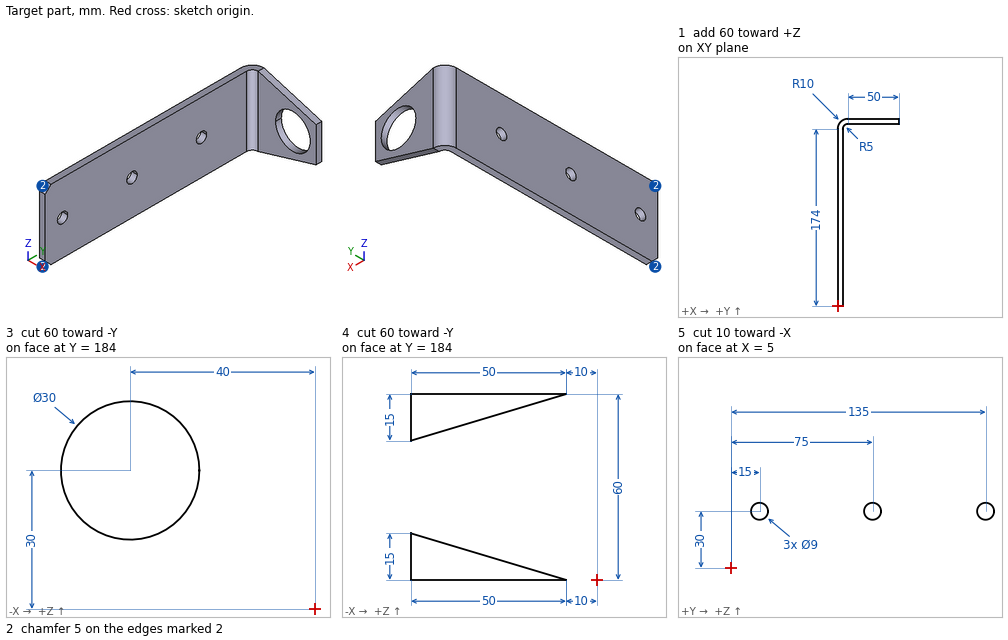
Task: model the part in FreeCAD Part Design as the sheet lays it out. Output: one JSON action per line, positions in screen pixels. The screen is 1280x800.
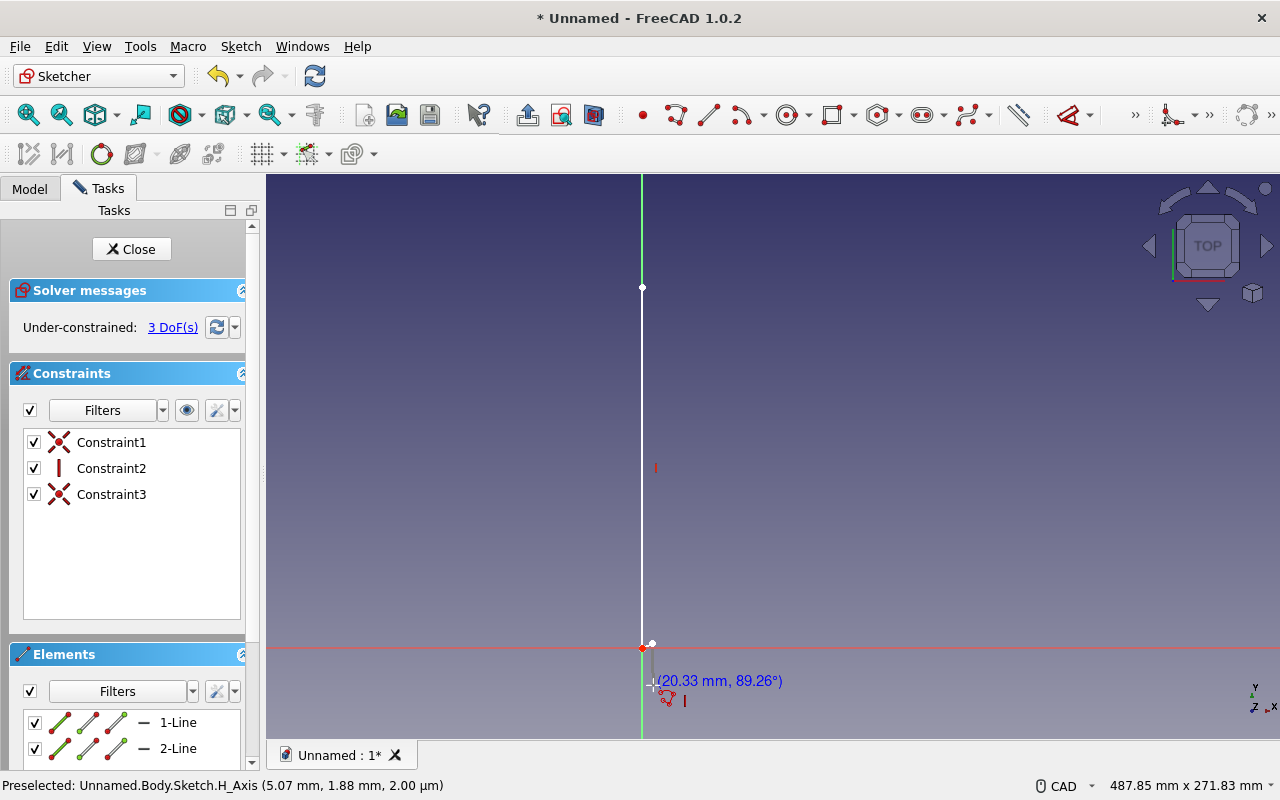
{"action": "scroll", "coordinate": [653, 287], "scroll_direction": "up", "scroll_amount": 3}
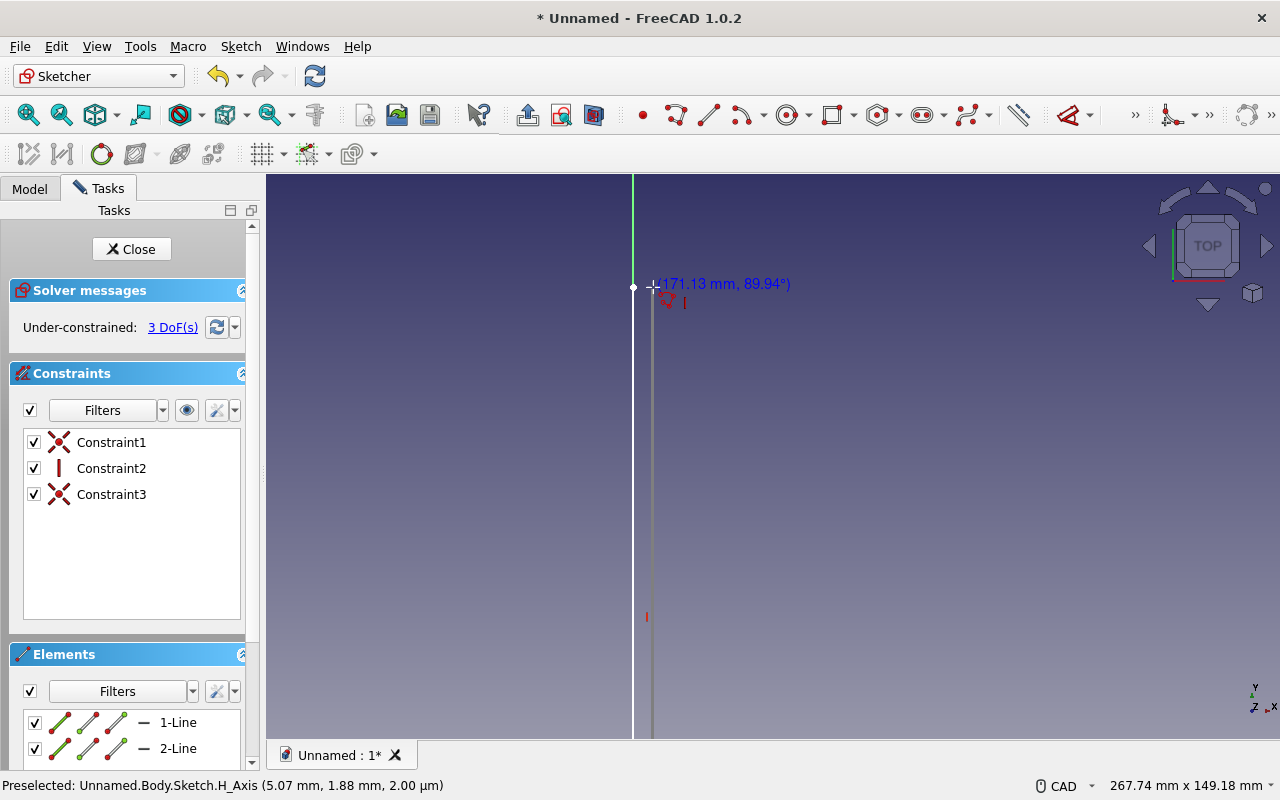
{"action": "left_click", "coordinate": [652, 286]}
{"action": "right_click", "coordinate": [652, 286]}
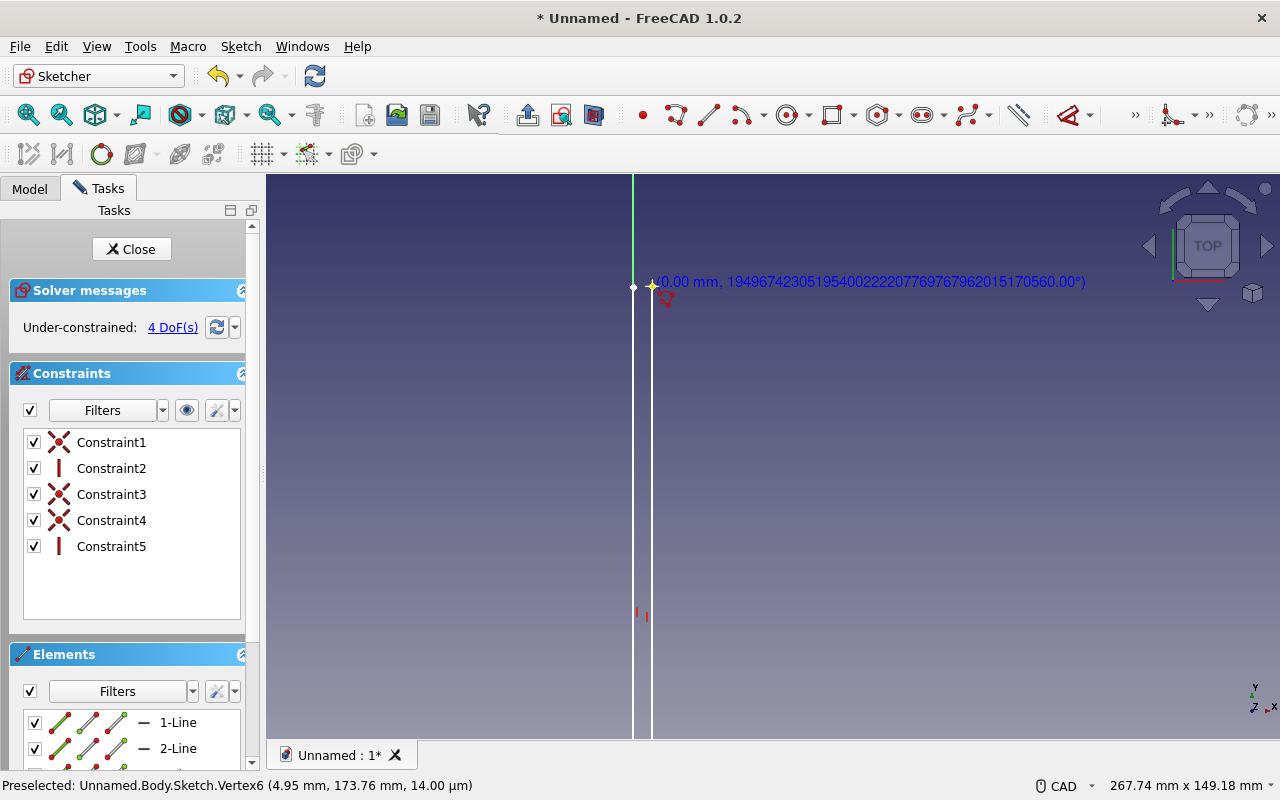
{"action": "left_click", "coordinate": [671, 267]}
{"action": "left_click", "coordinate": [860, 267]}
{"action": "left_click", "coordinate": [860, 248]}
{"action": "left_click", "coordinate": [671, 248]}
{"action": "right_click", "coordinate": [671, 248]}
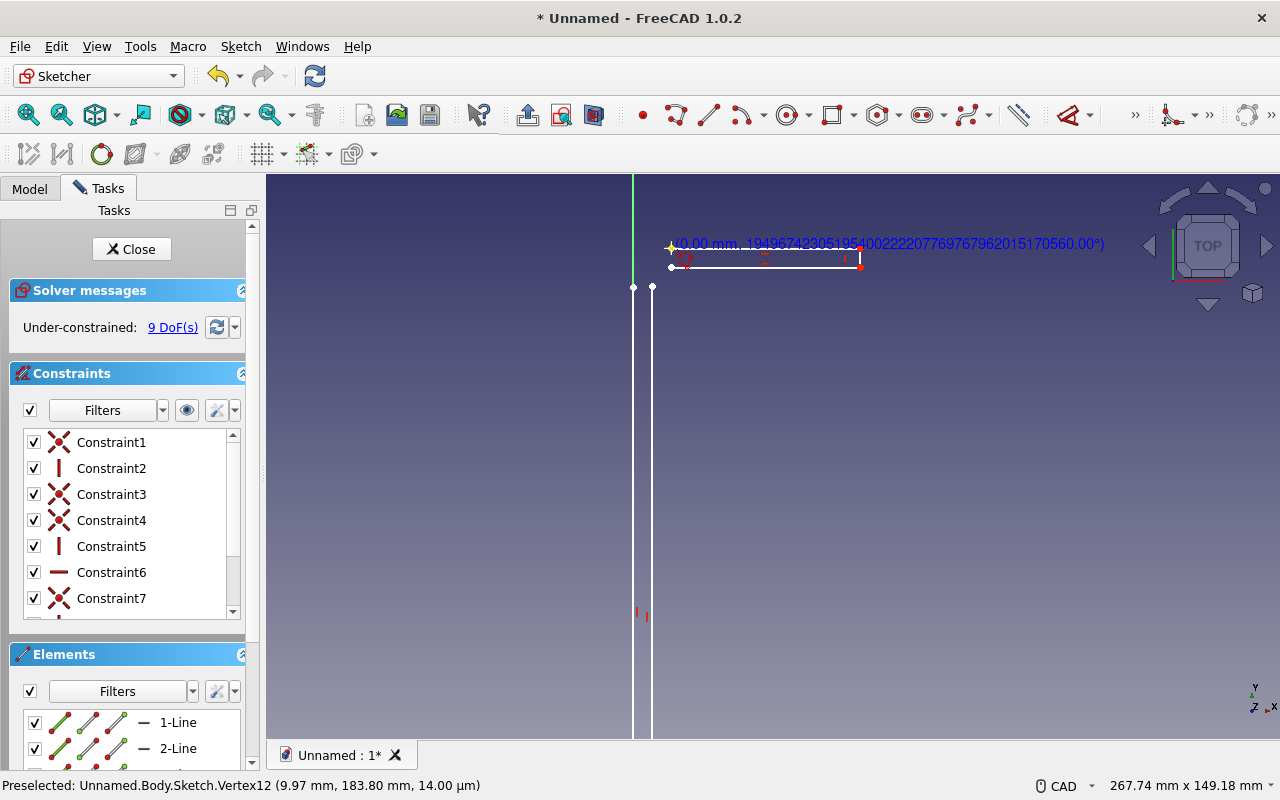
{"action": "key", "text": "g 3 a"}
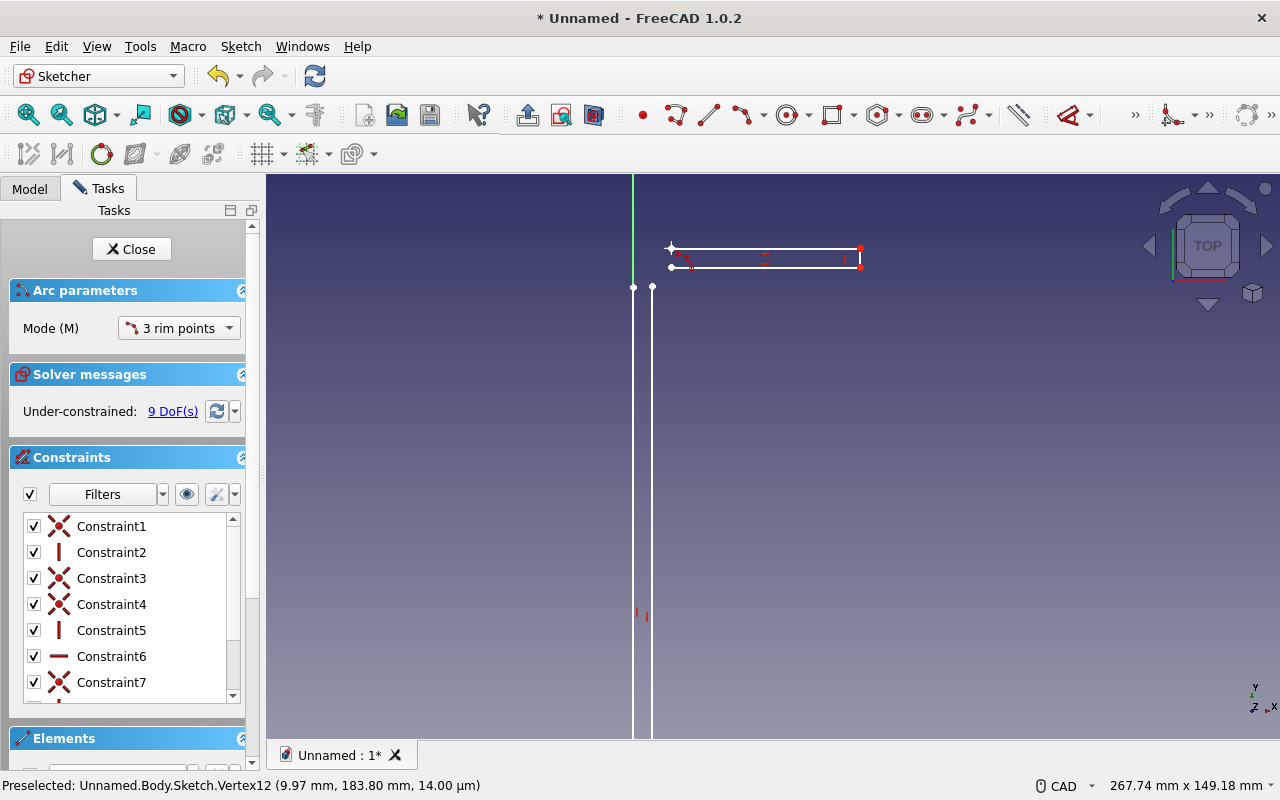
{"action": "left_click", "coordinate": [652, 287]}
{"action": "left_click", "coordinate": [671, 268]}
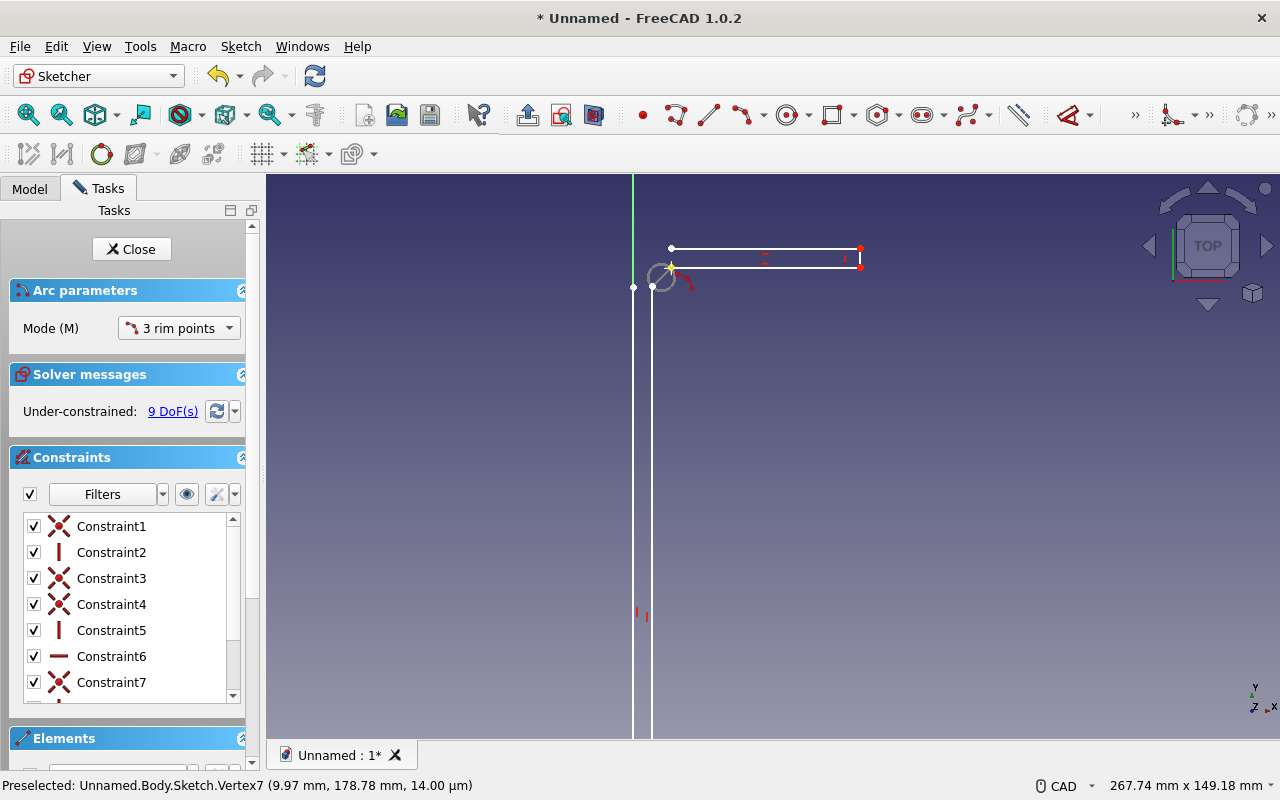
{"action": "scroll", "coordinate": [658, 273], "scroll_direction": "up", "scroll_amount": 6}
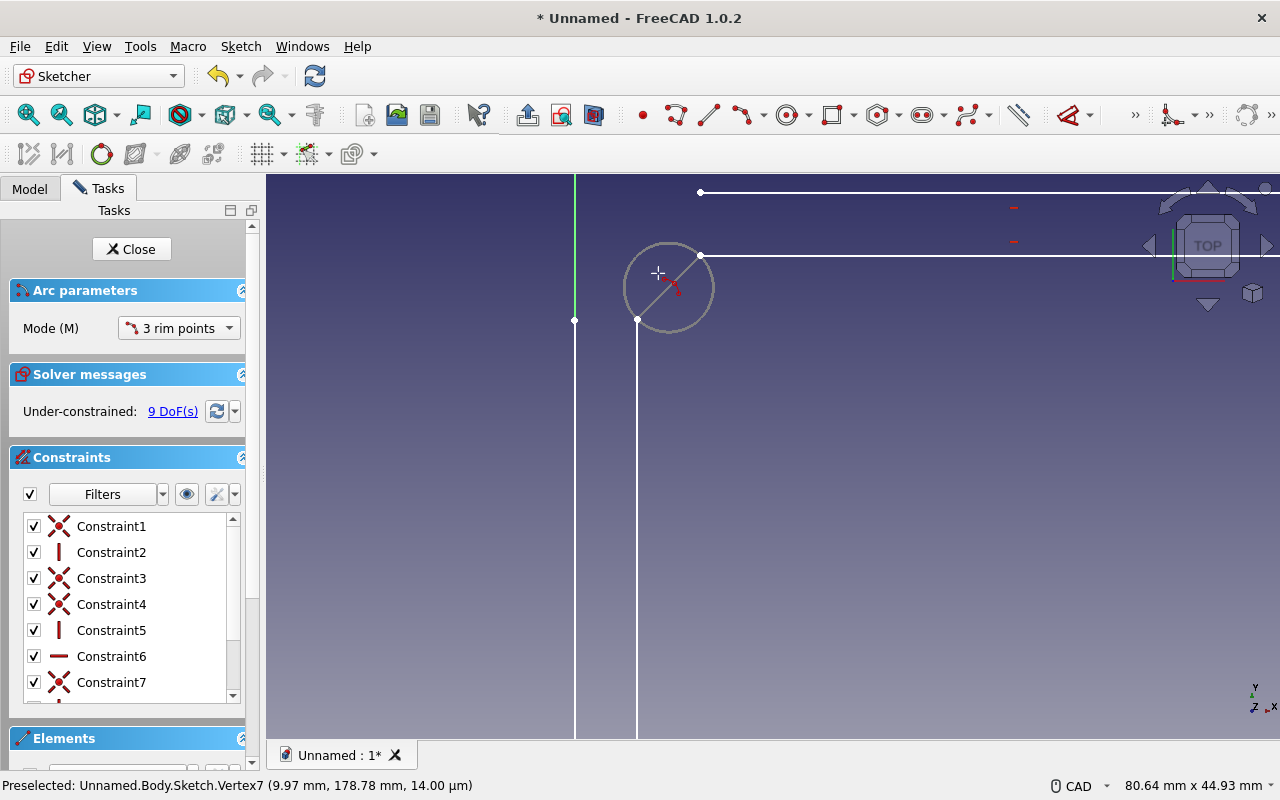
{"action": "left_click", "coordinate": [656, 272]}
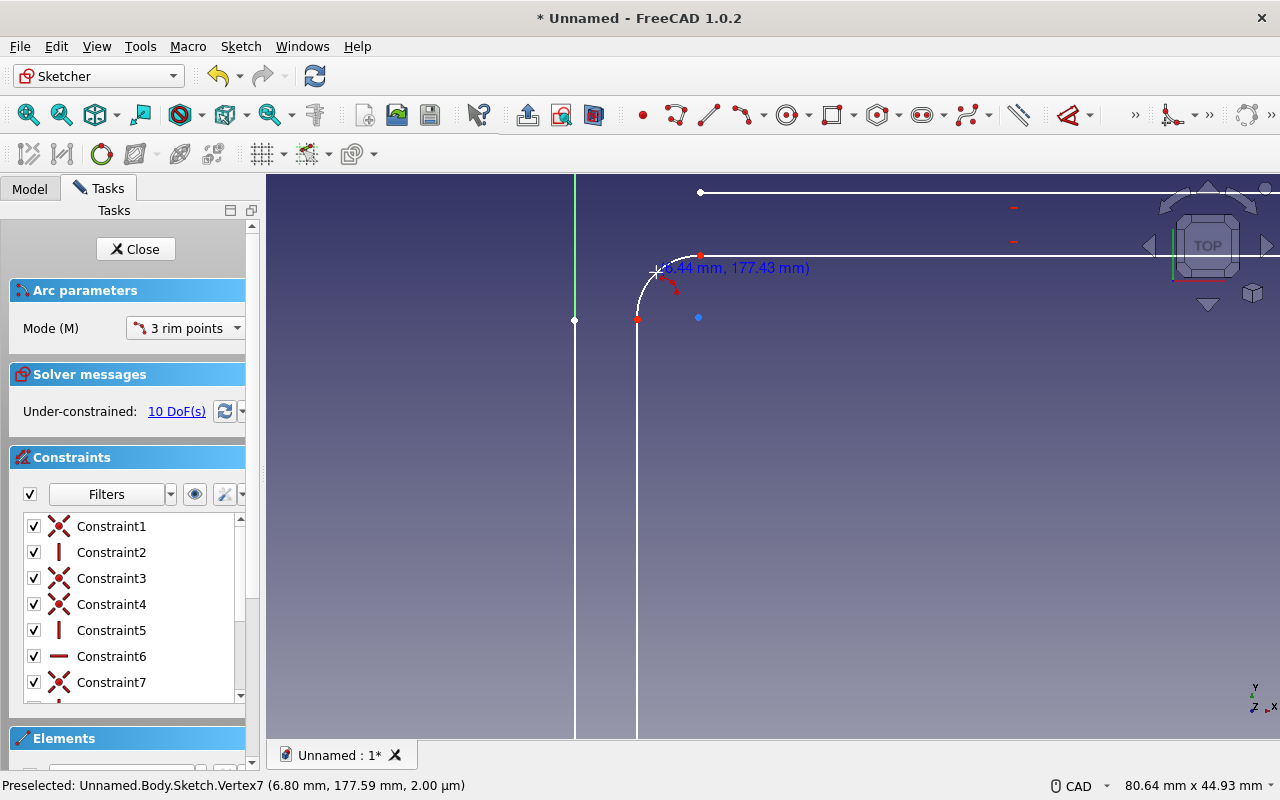
{"action": "scroll", "coordinate": [655, 280], "scroll_direction": "down", "scroll_amount": 9}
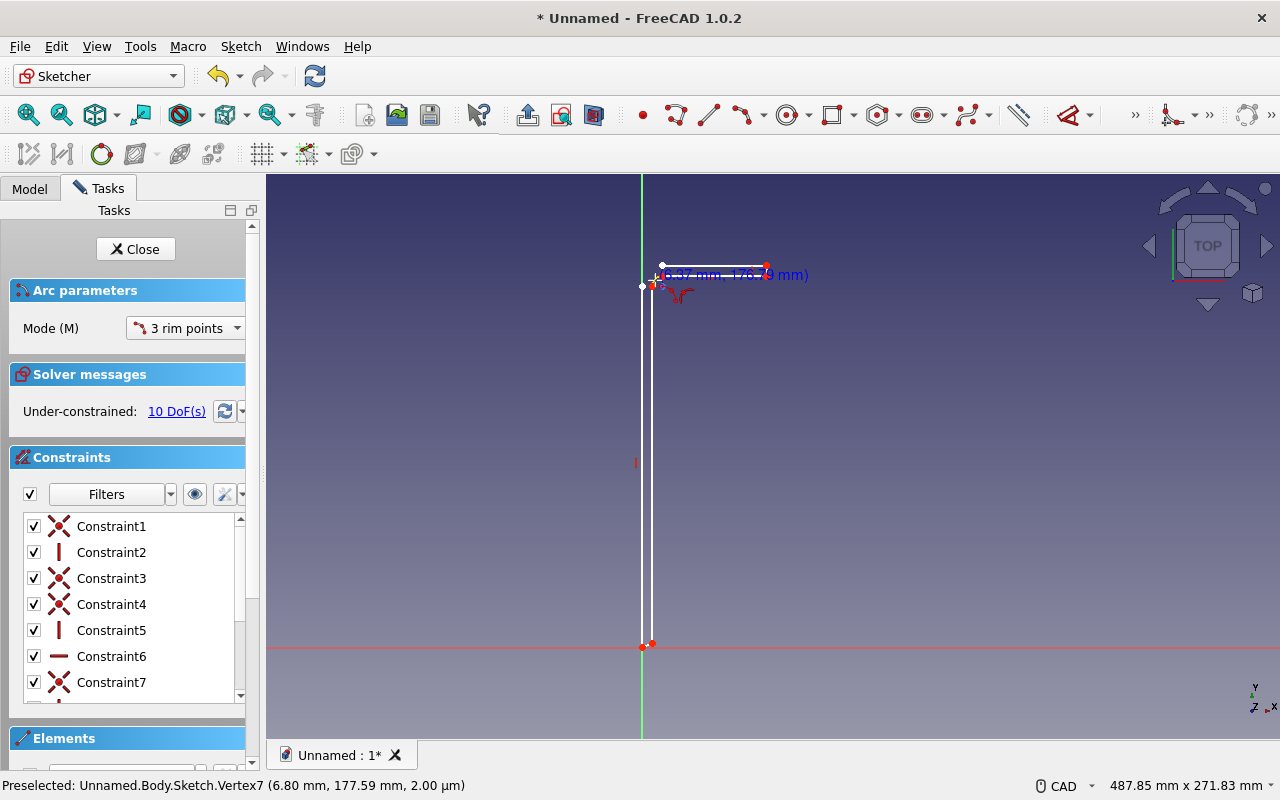
{"action": "scroll", "coordinate": [663, 265], "scroll_direction": "up", "scroll_amount": 3}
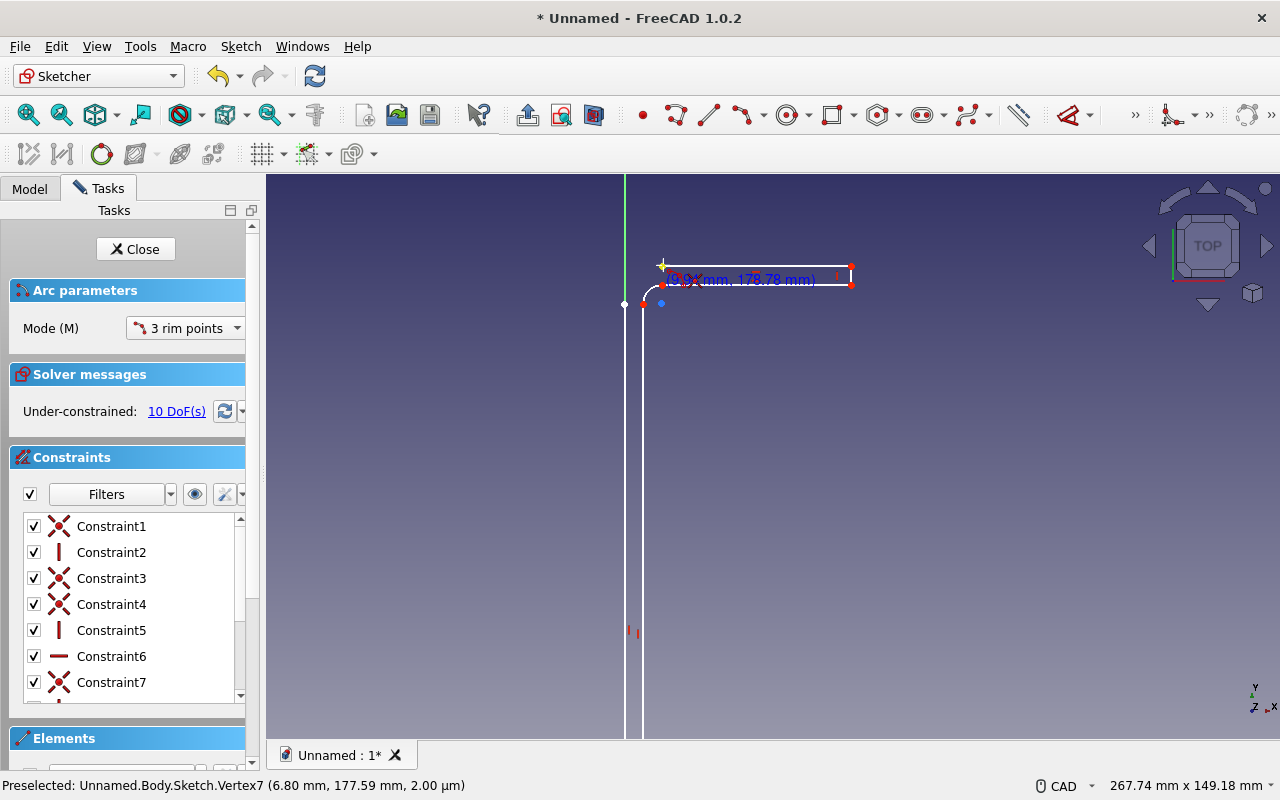
{"action": "left_click", "coordinate": [662, 266]}
{"action": "left_click", "coordinate": [625, 305]}